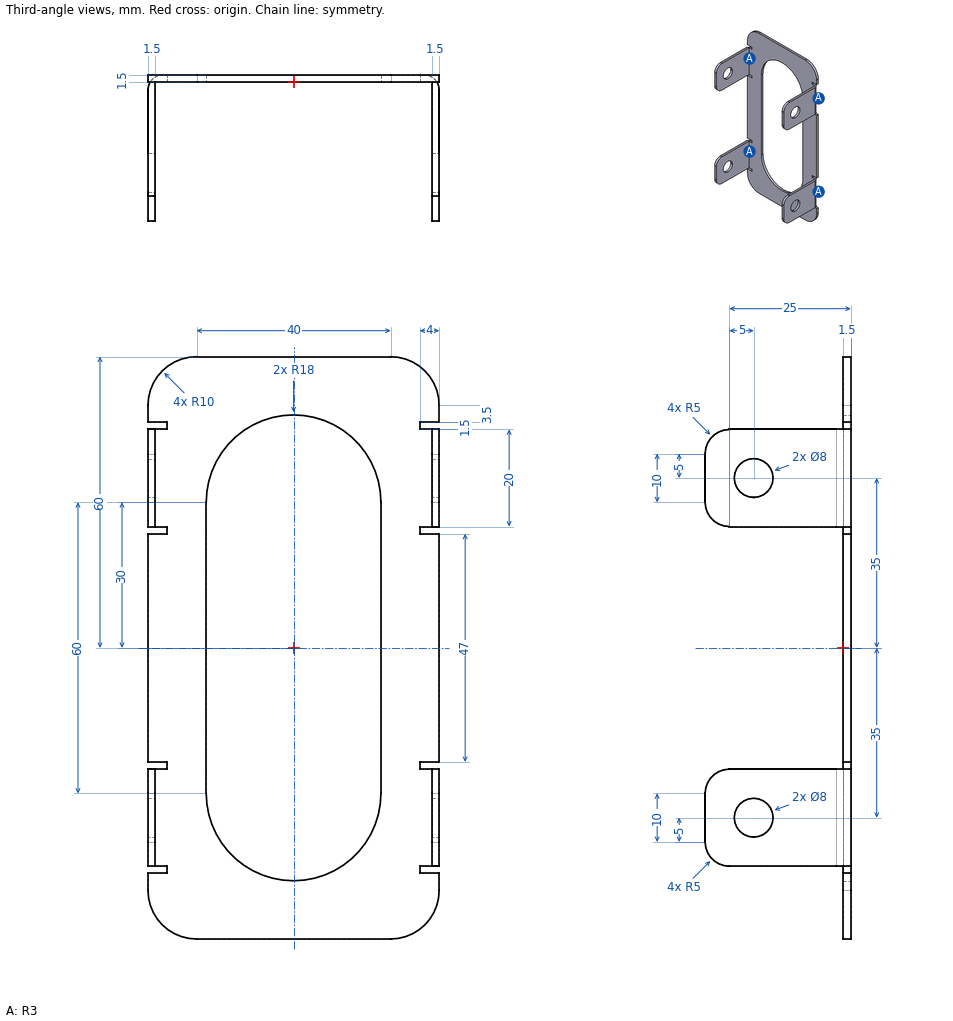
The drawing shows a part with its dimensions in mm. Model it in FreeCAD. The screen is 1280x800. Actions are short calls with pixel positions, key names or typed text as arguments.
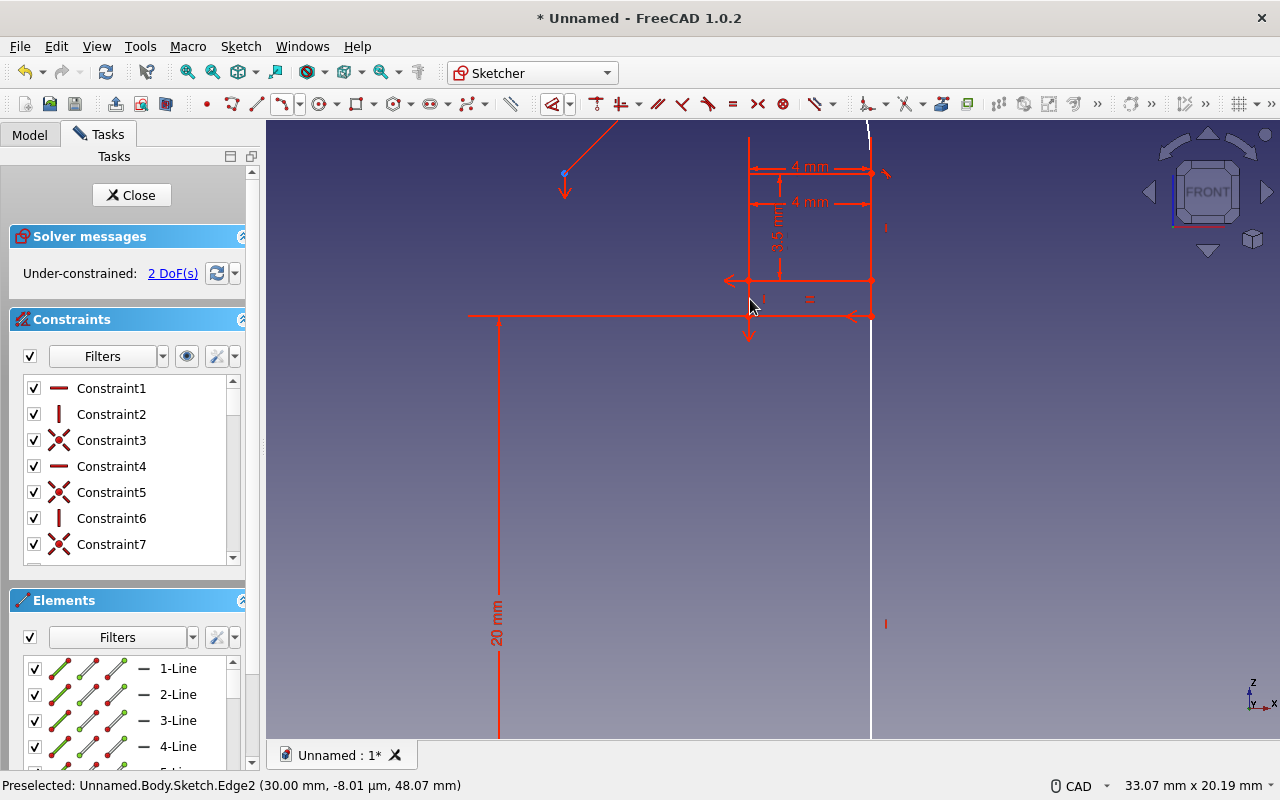
click(749, 299)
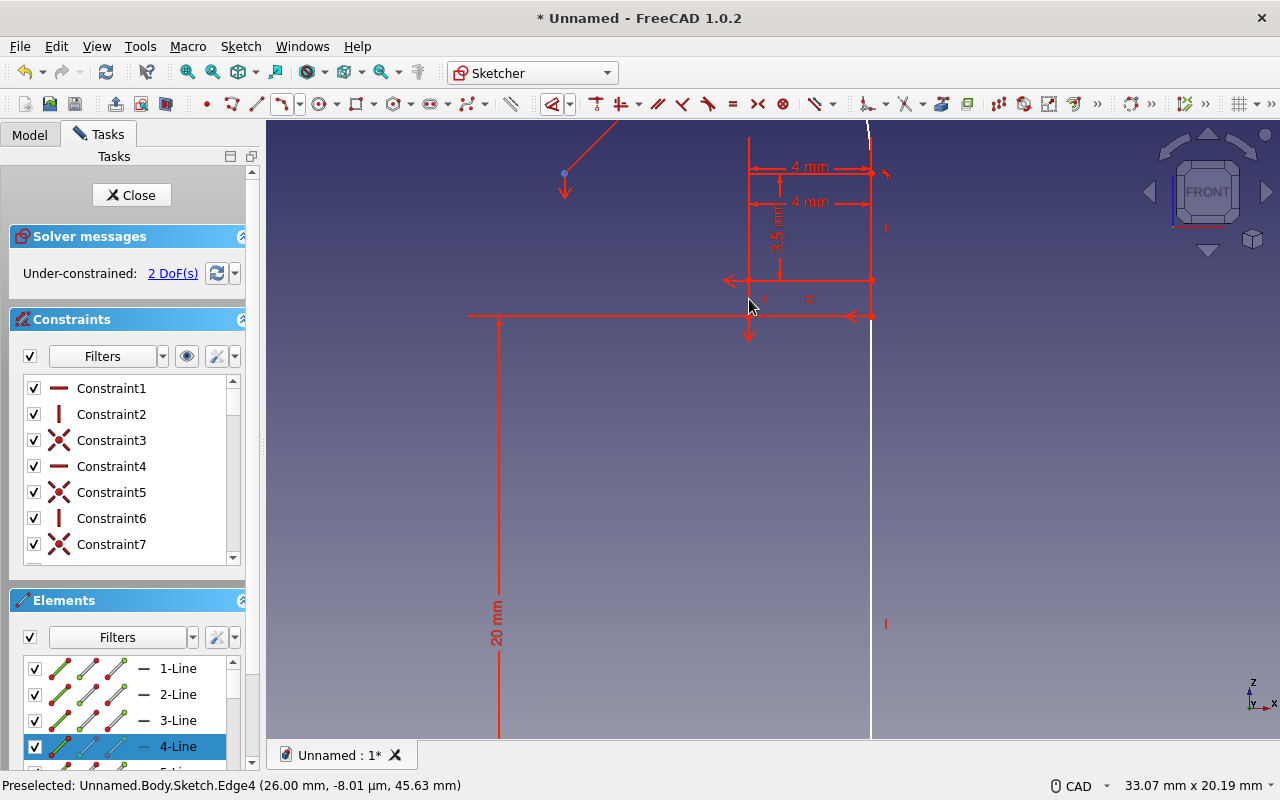
click(570, 104)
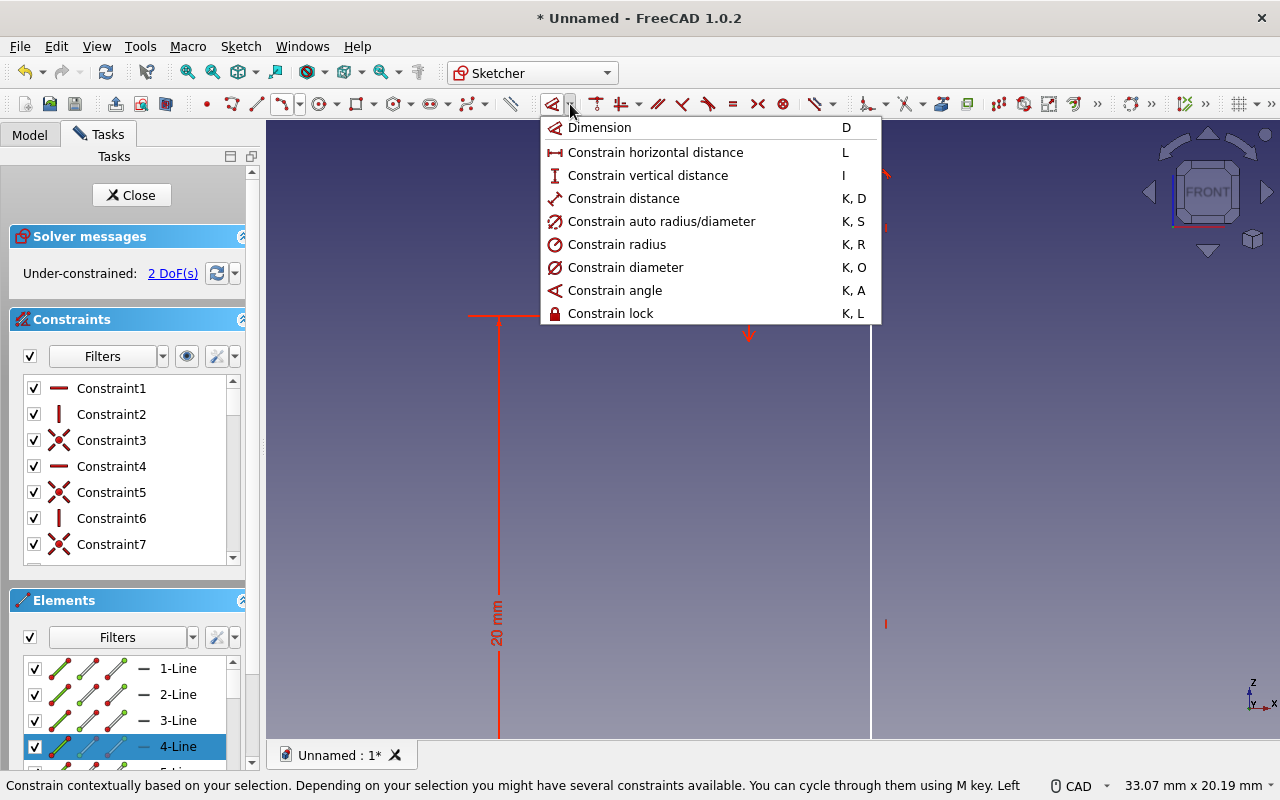
click(711, 176)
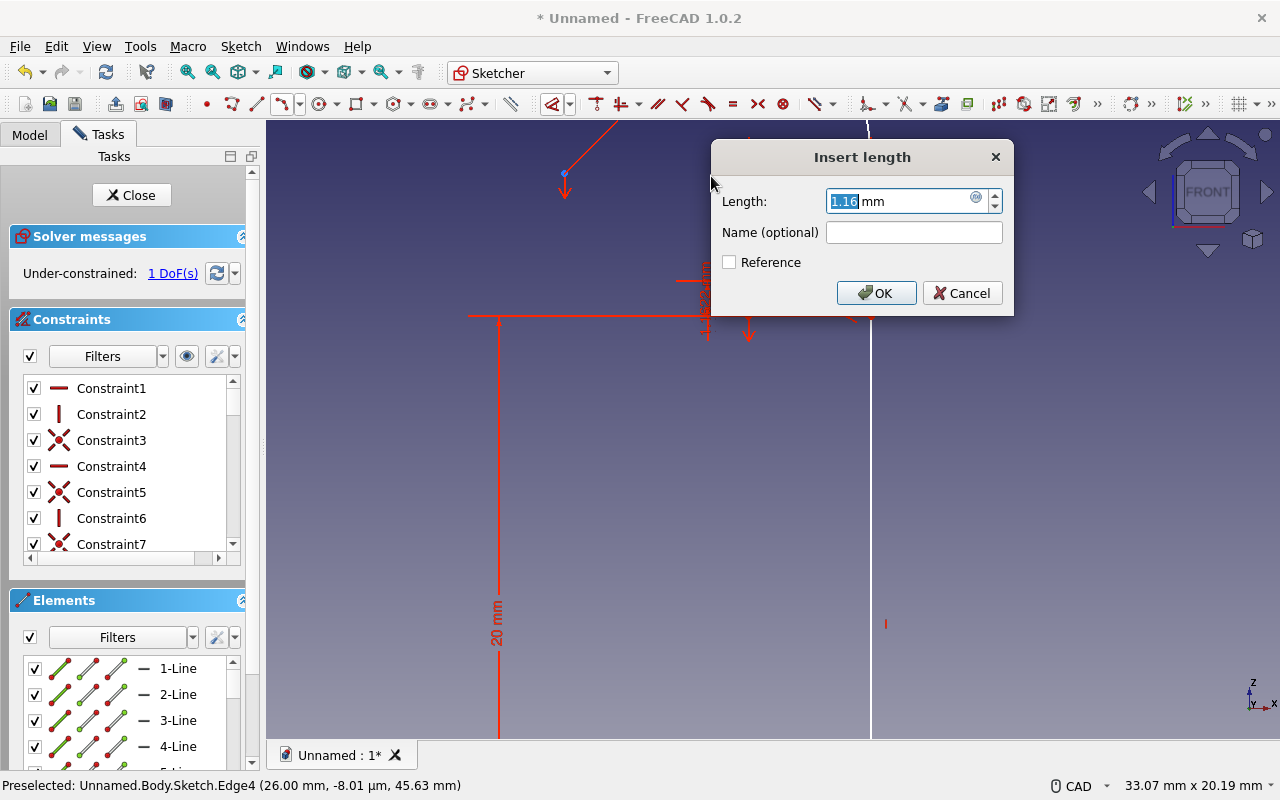
text(1.5)
key(Return)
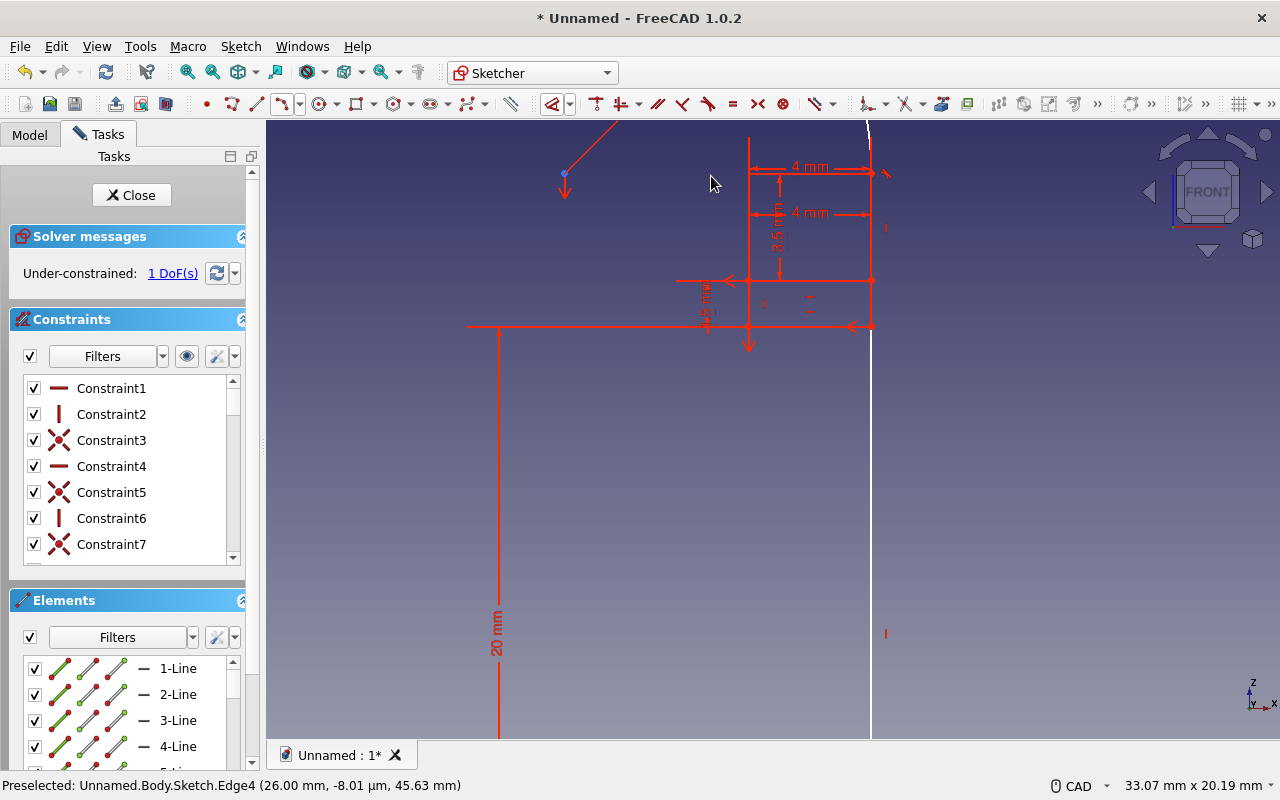
scroll(798, 271, down, 11)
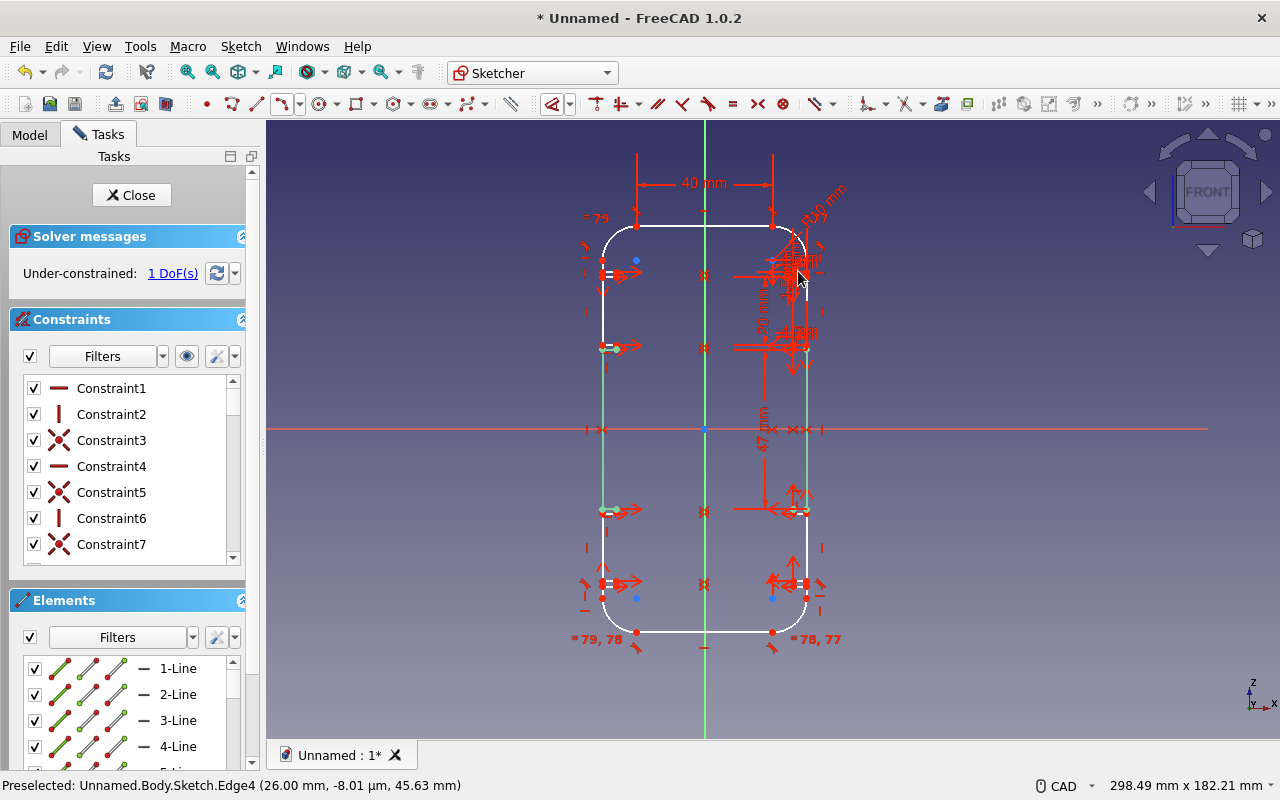
click(637, 226)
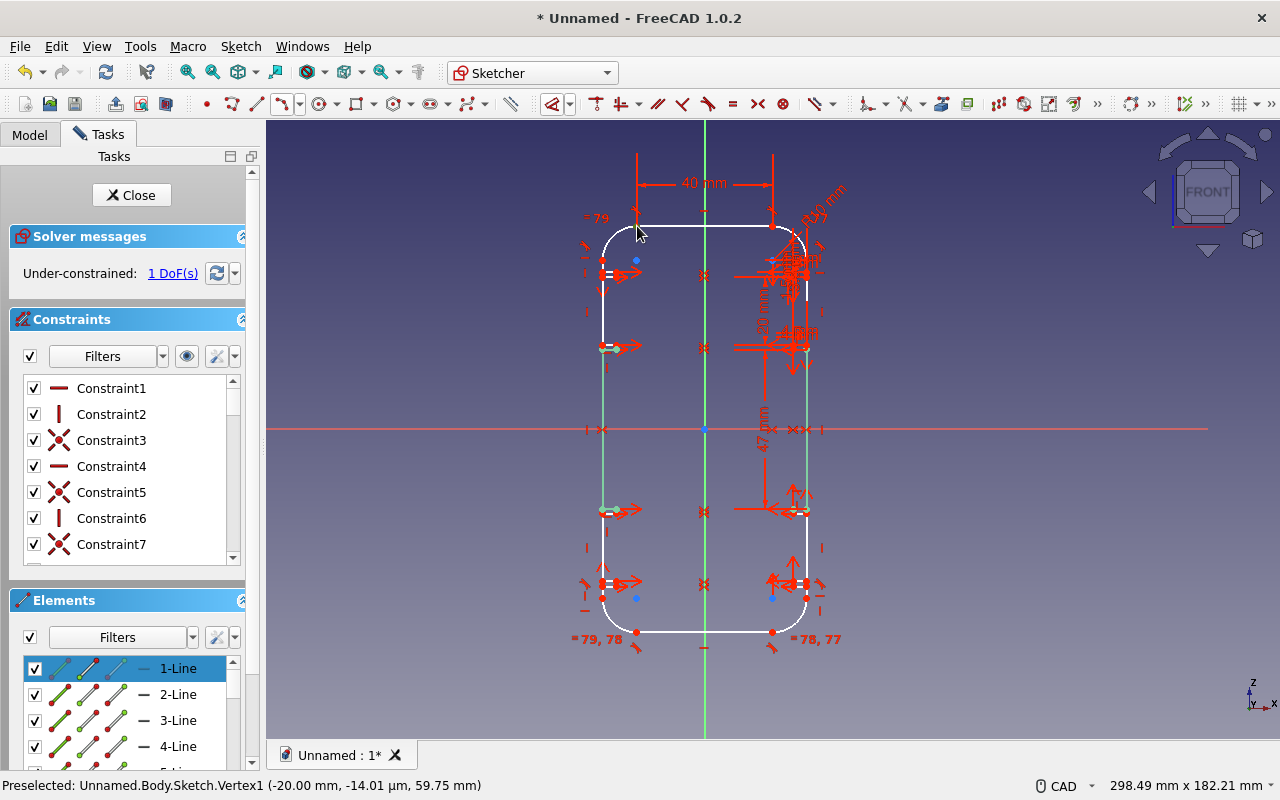
key(i)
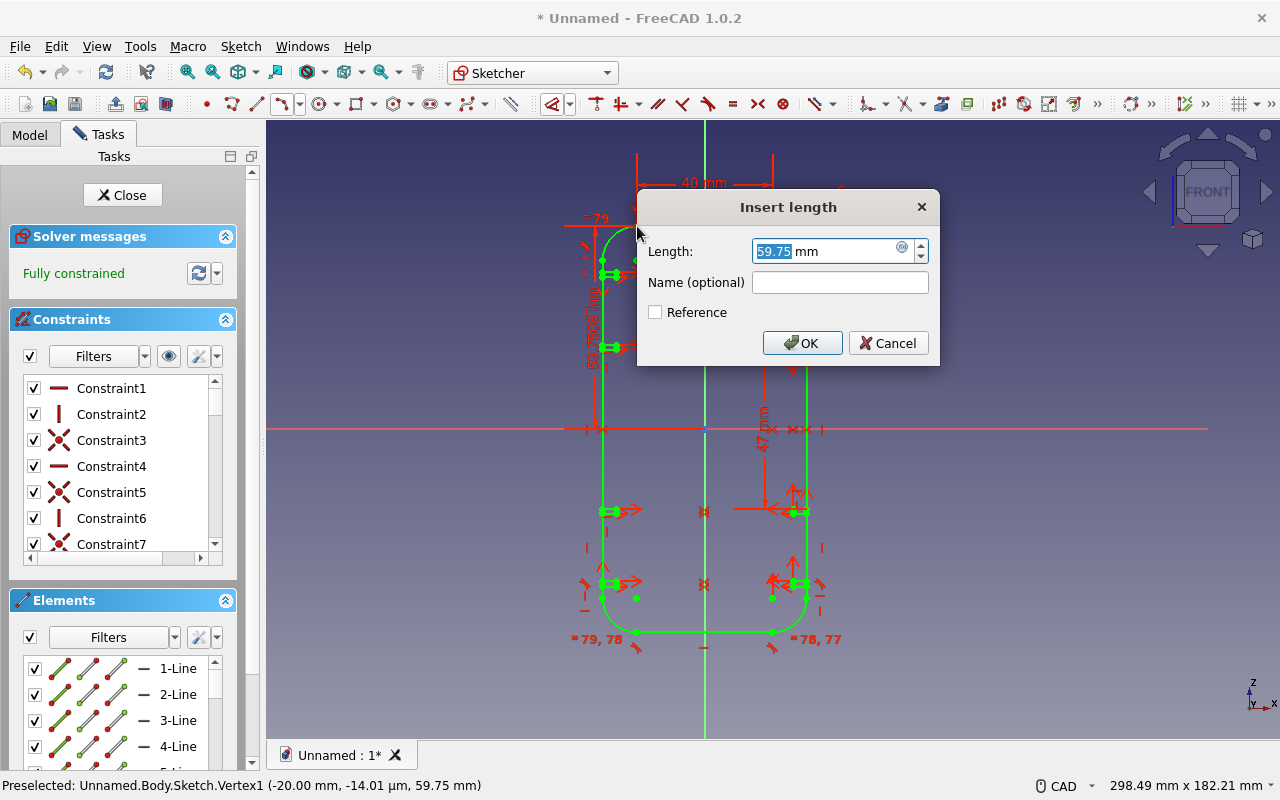
text(60)
key(Return)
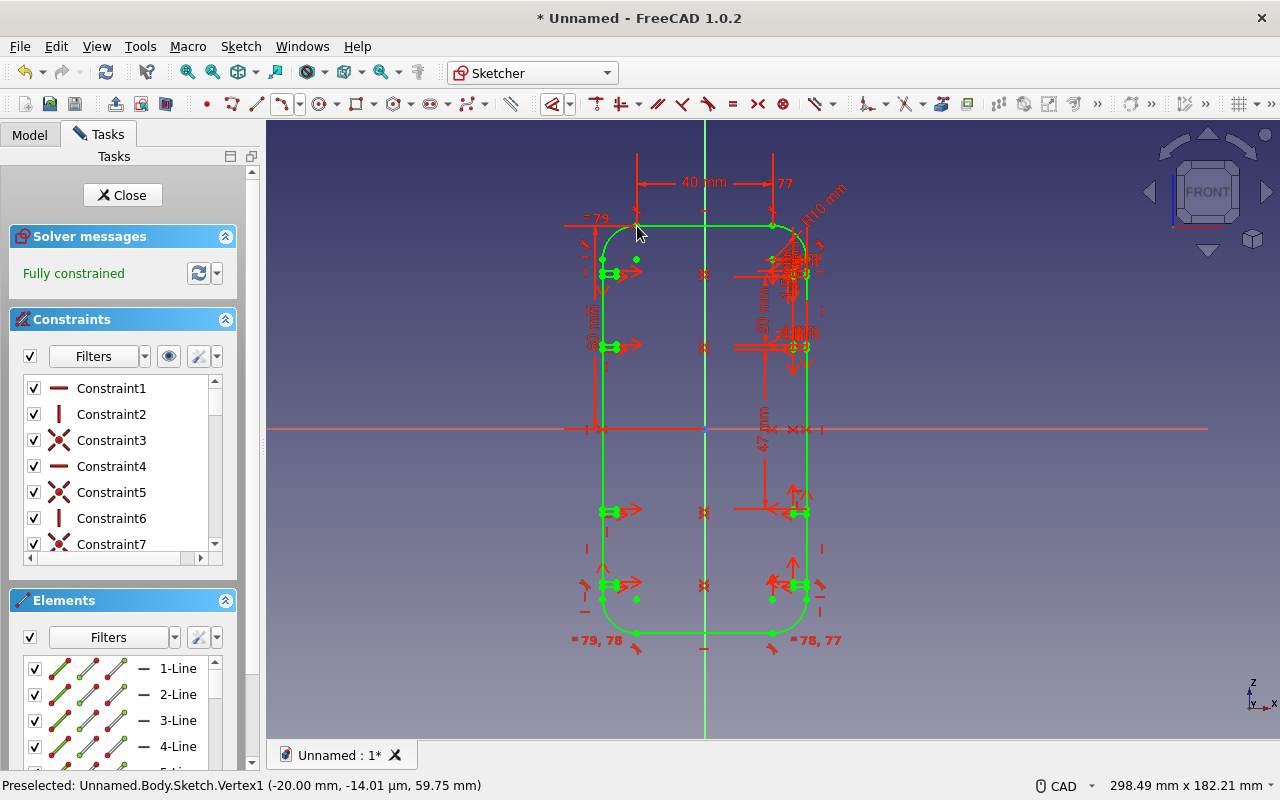
click(123, 195)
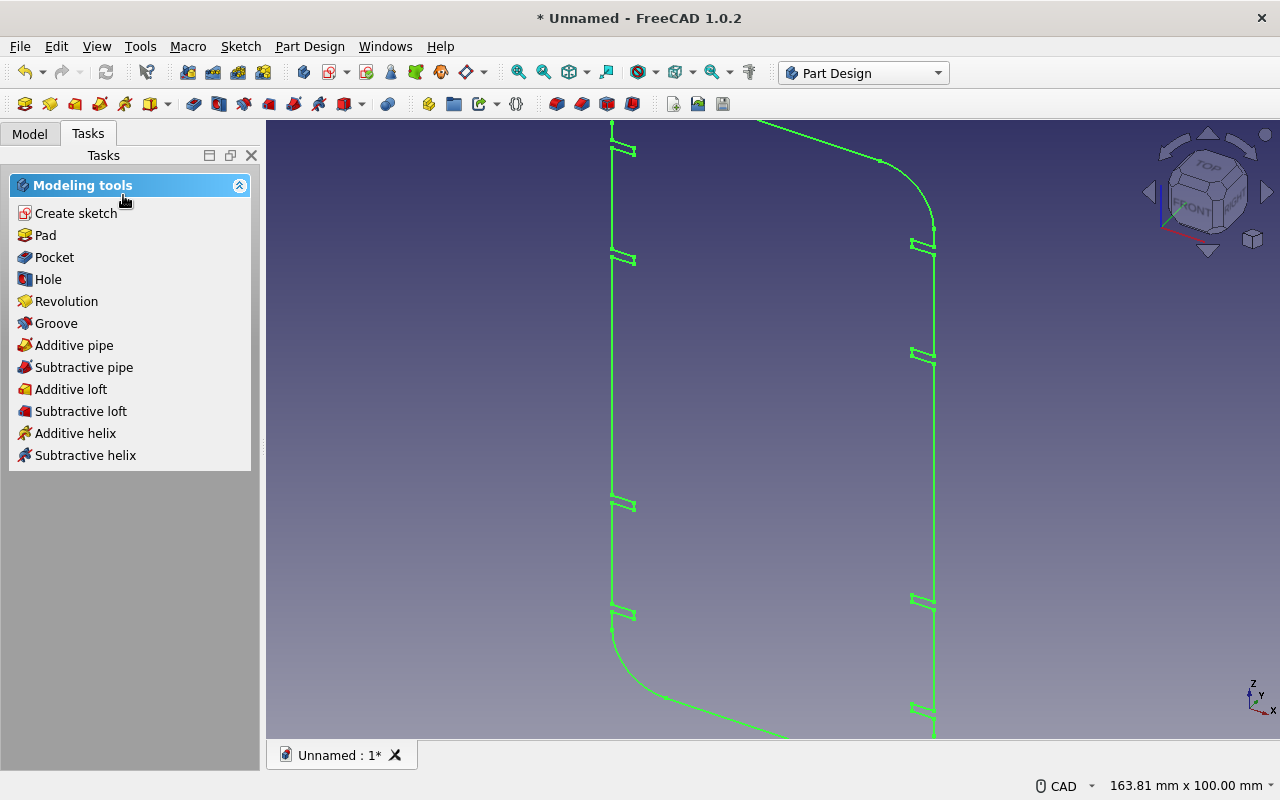
click(25, 104)